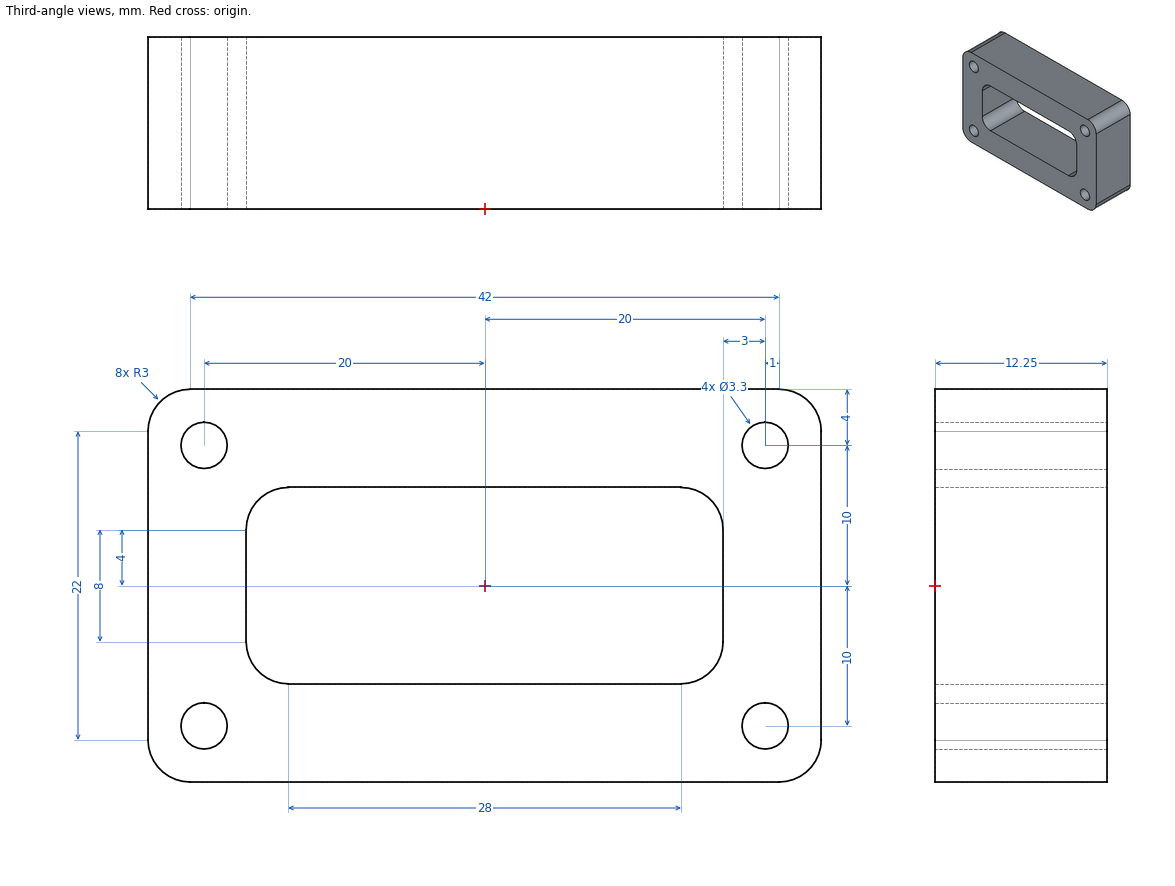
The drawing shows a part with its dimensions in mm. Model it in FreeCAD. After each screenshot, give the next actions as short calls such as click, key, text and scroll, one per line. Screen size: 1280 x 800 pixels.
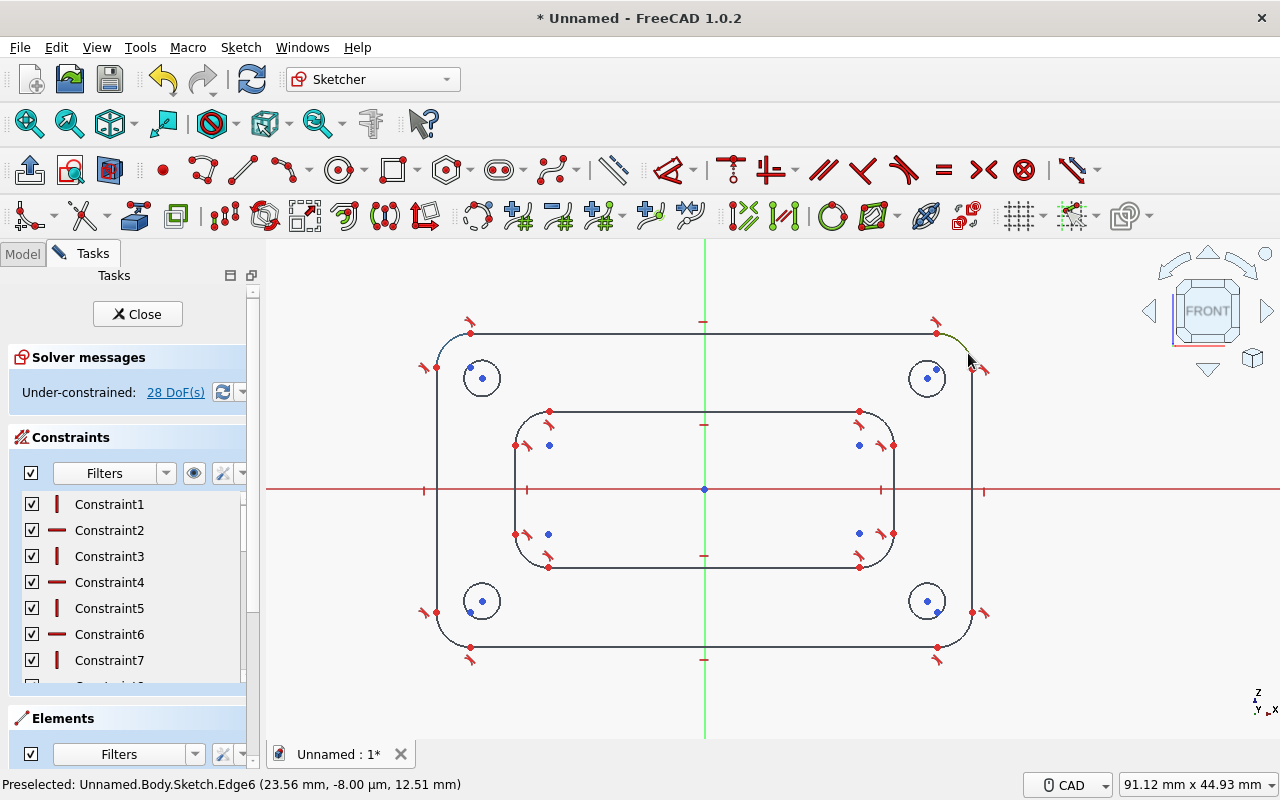
click(954, 643)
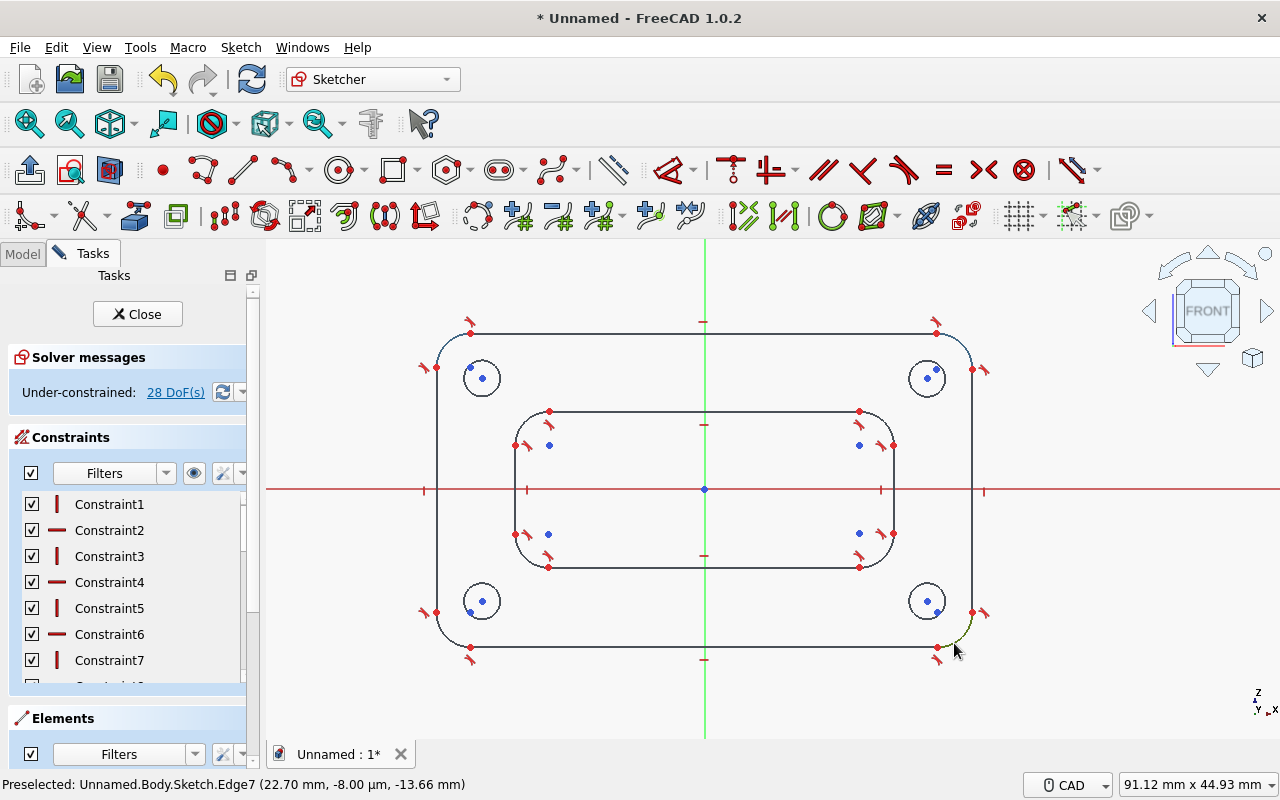
click(440, 628)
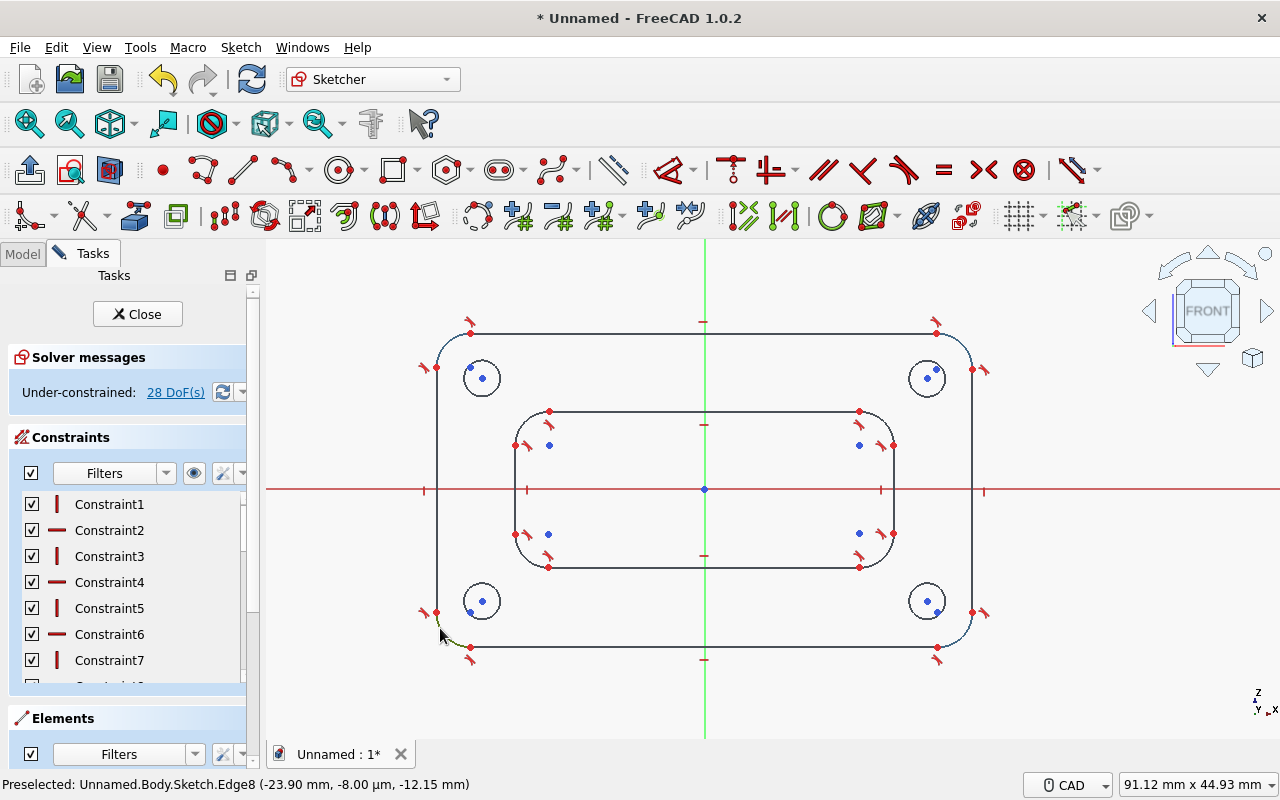
click(519, 550)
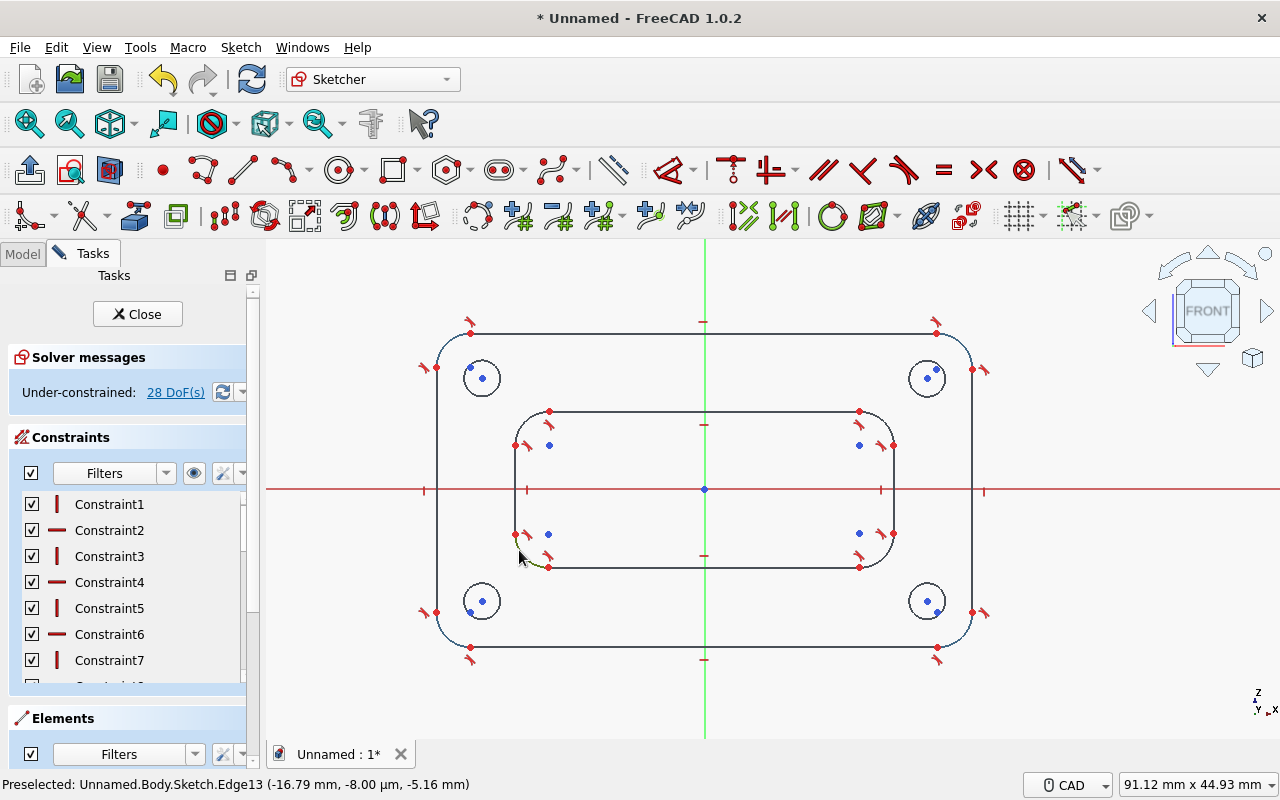
click(875, 564)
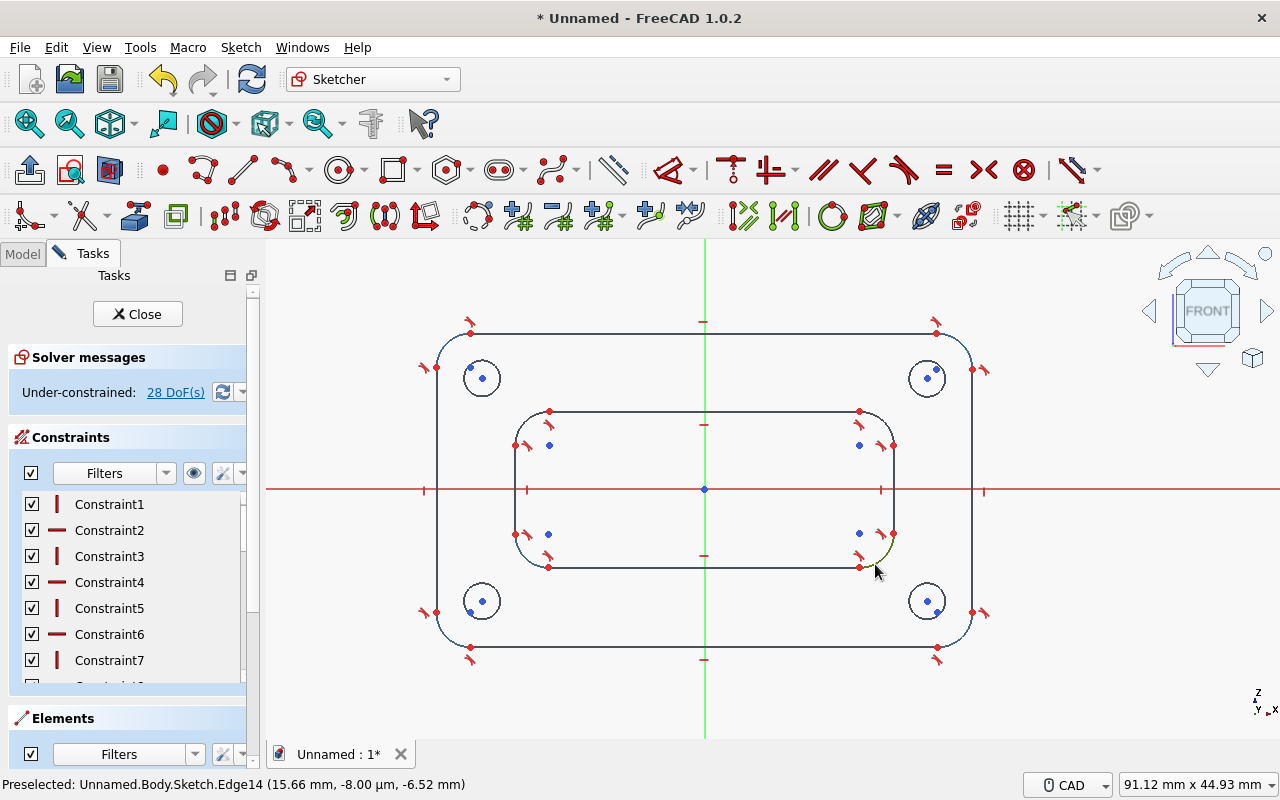
click(890, 431)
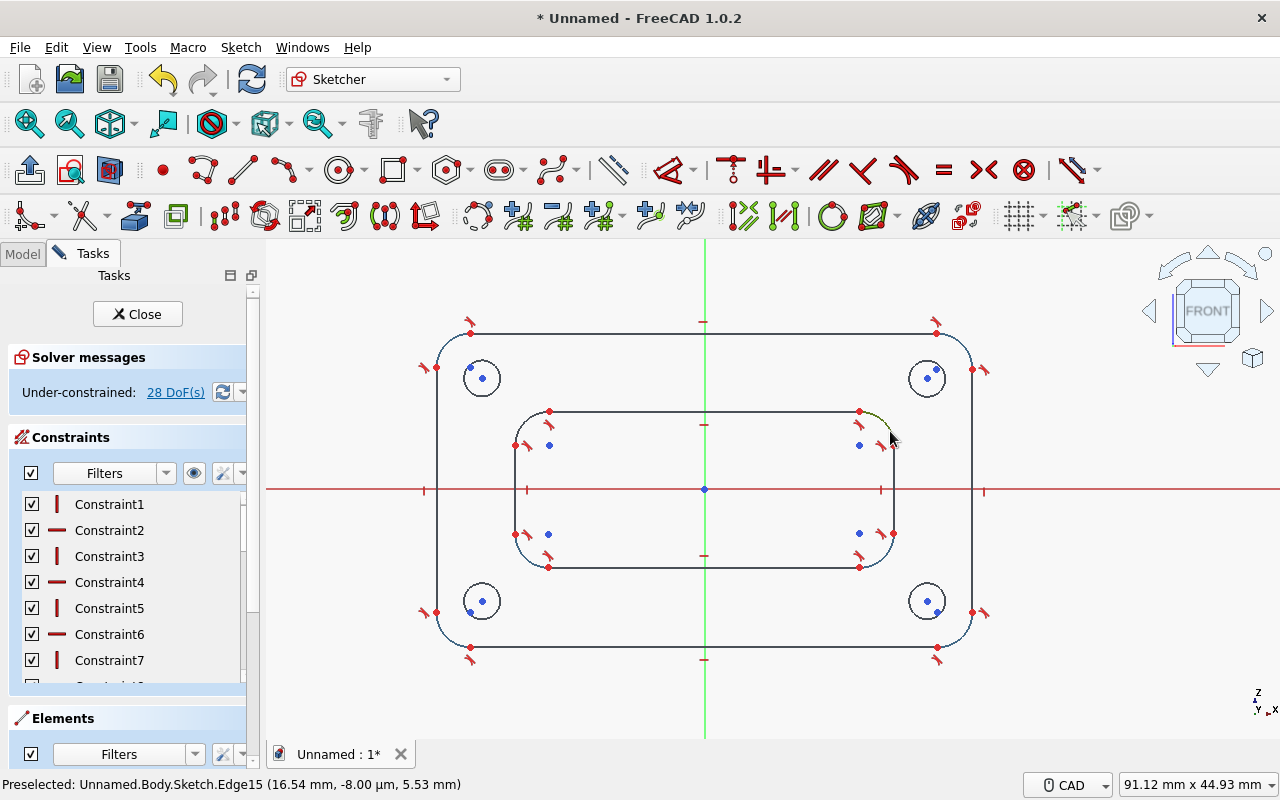
click(534, 416)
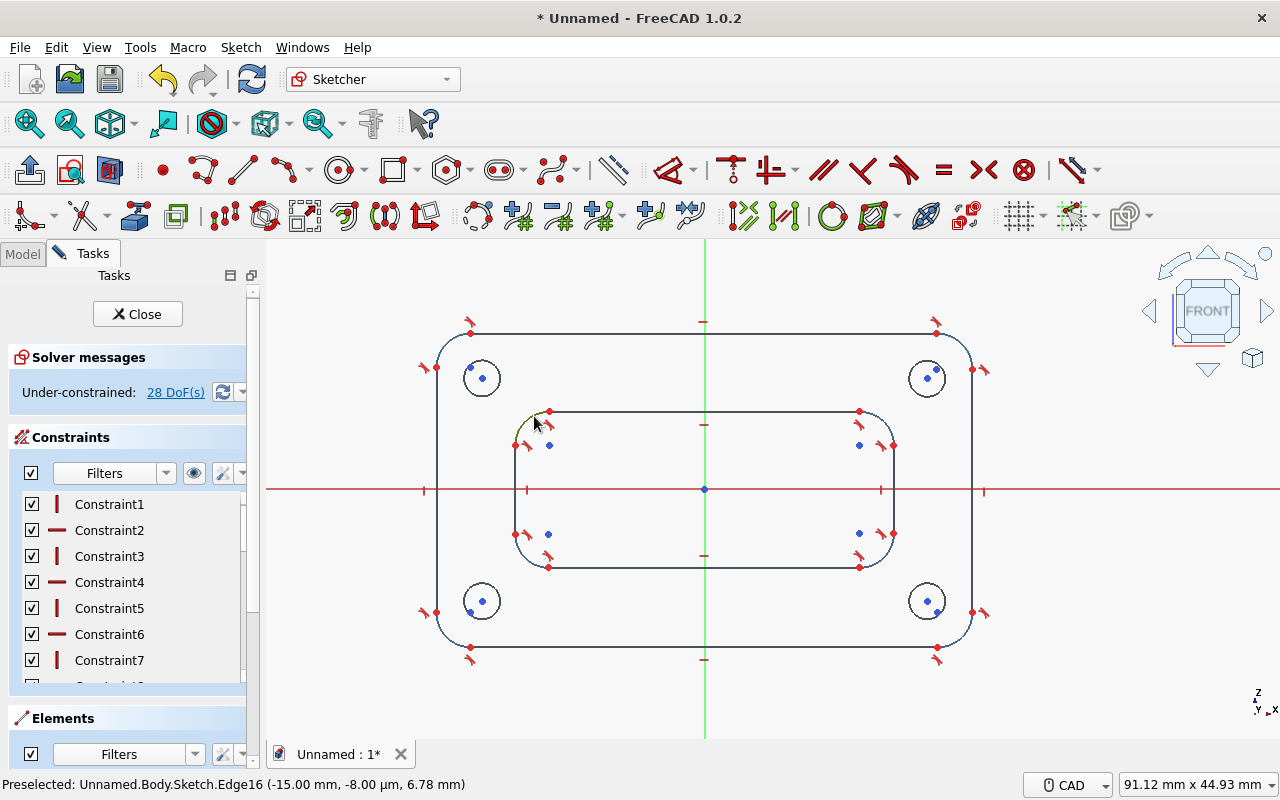
click(944, 170)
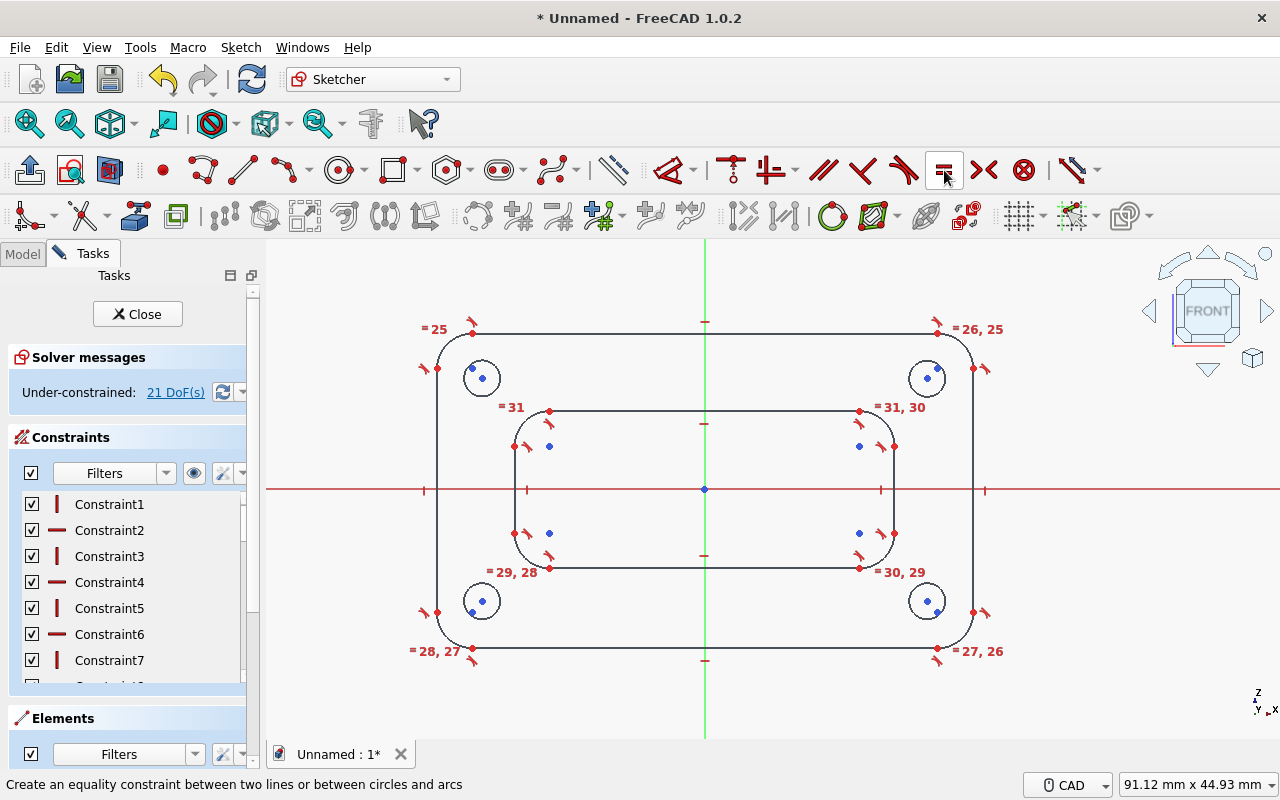
click(914, 366)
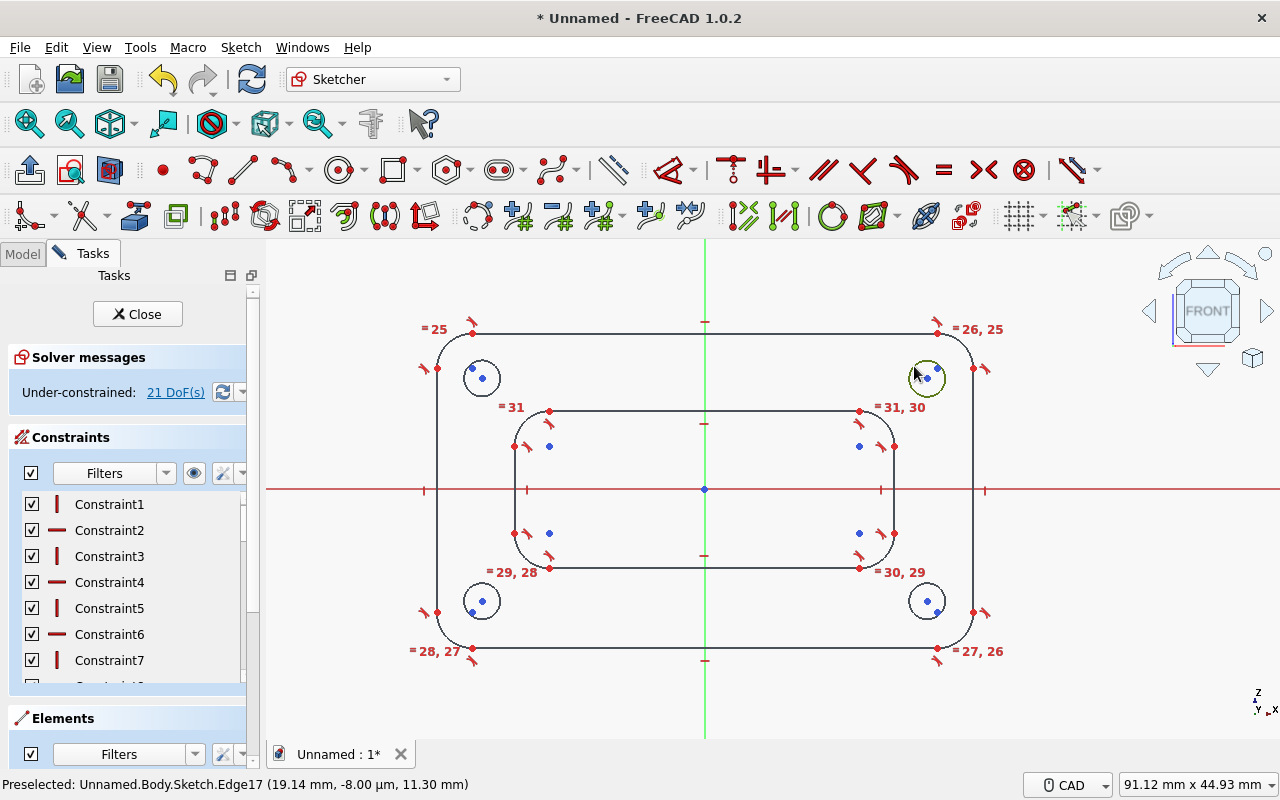
click(495, 366)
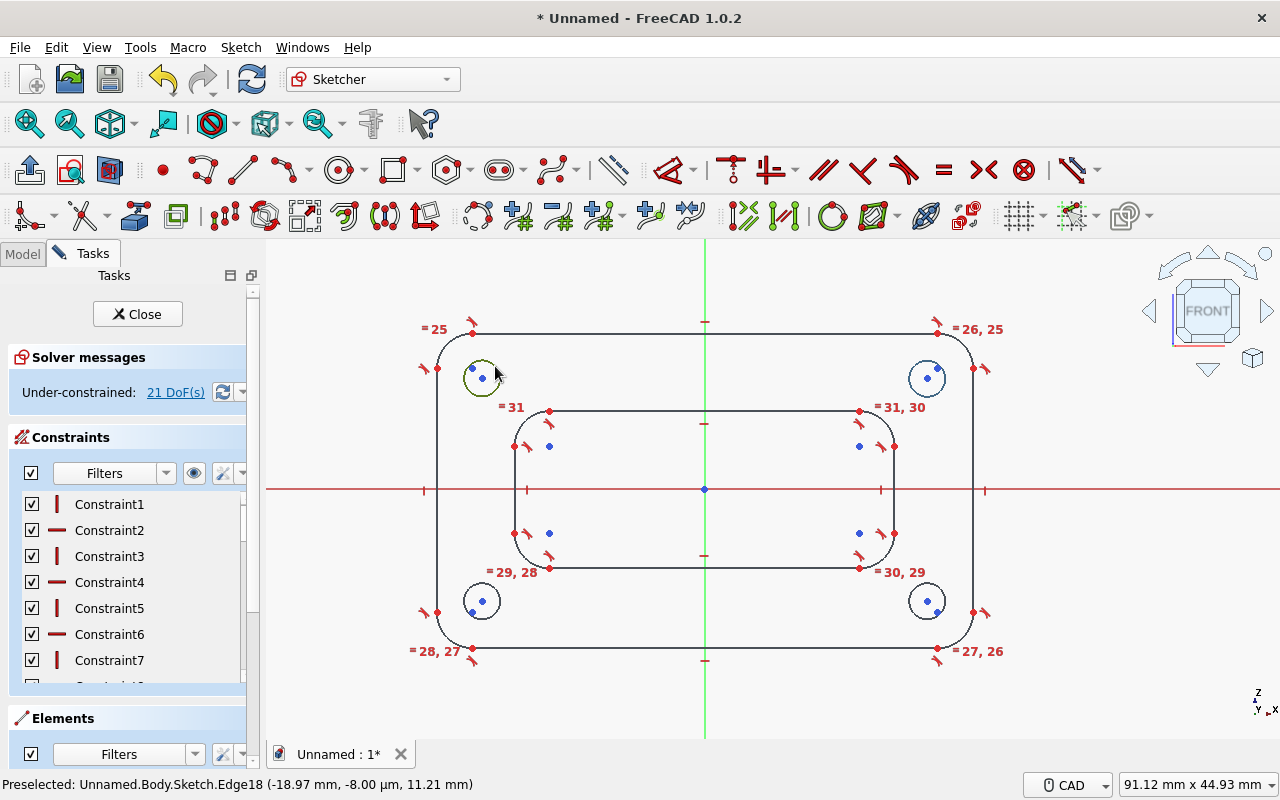
click(940, 588)